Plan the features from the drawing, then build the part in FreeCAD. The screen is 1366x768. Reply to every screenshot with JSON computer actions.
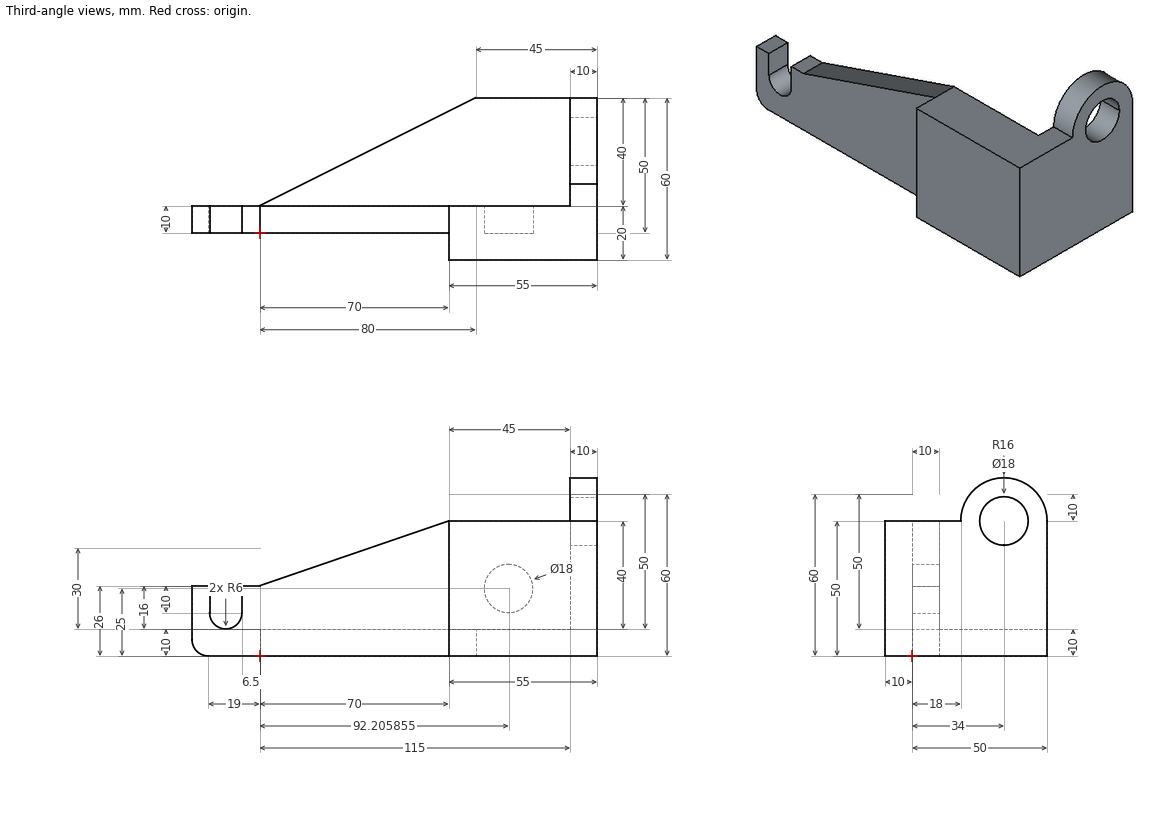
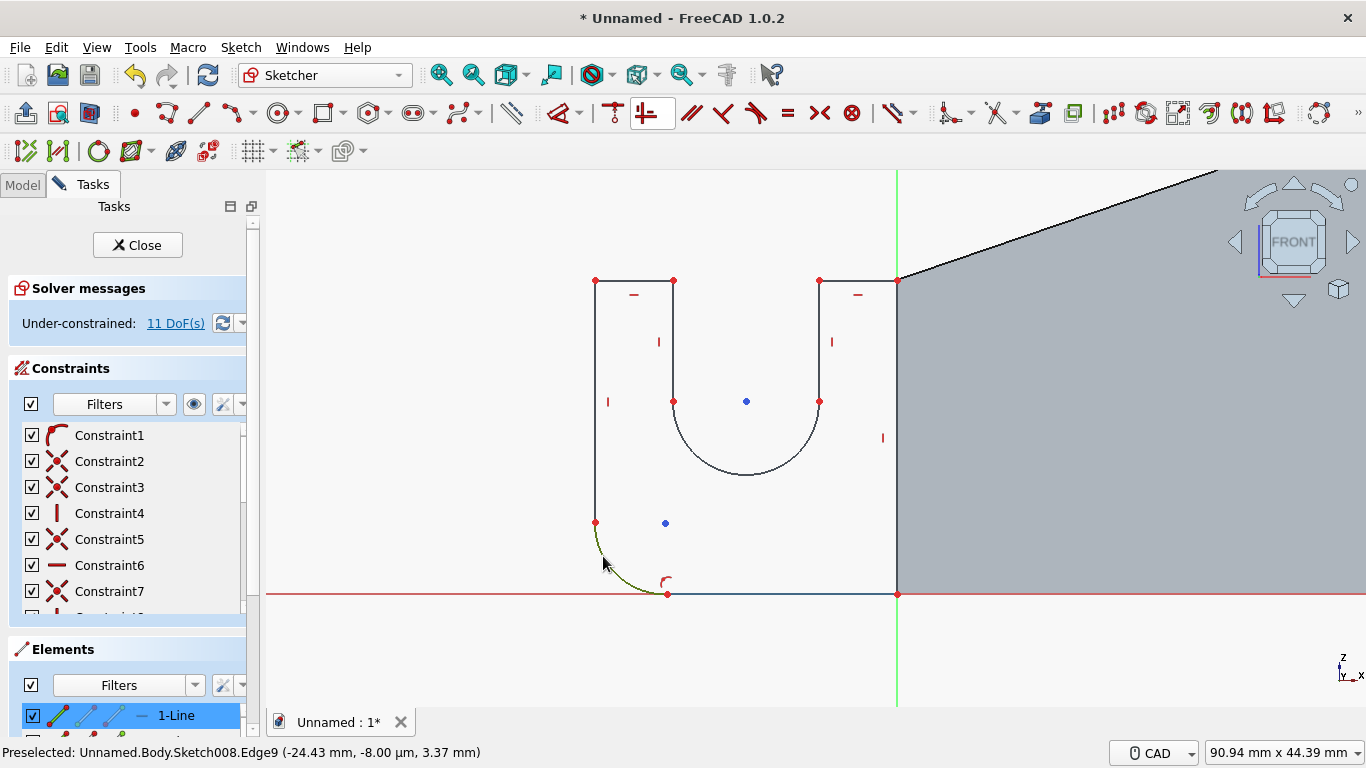
{"action": "left_click", "coordinate": [756, 114]}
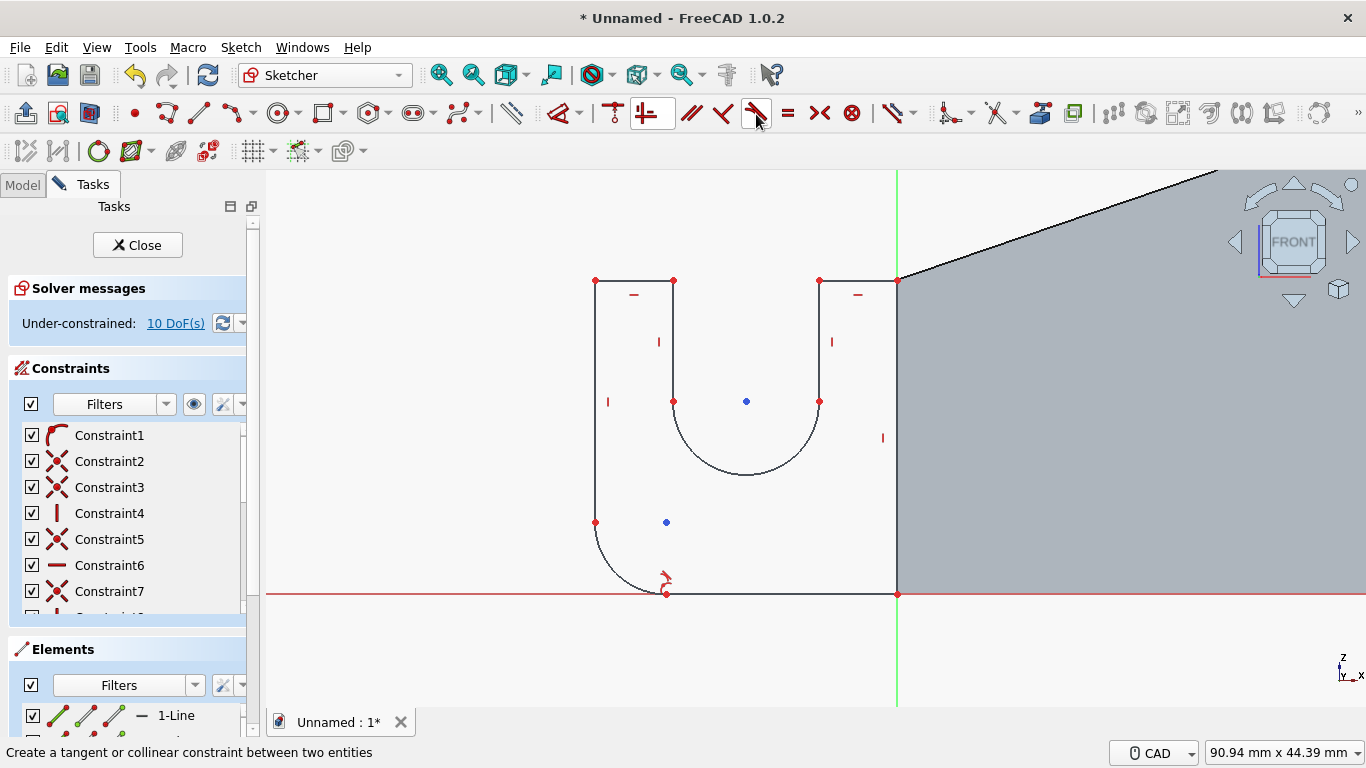
{"action": "left_click", "coordinate": [819, 317]}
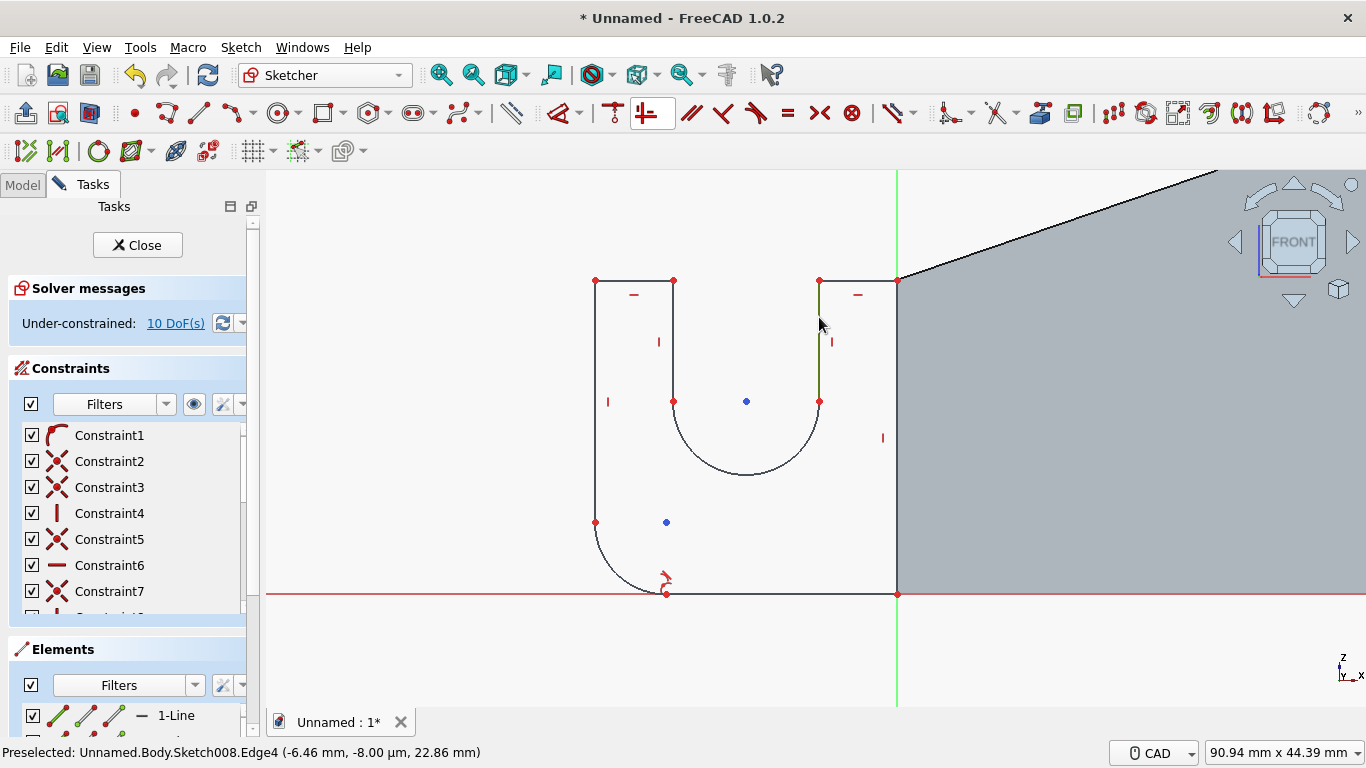
{"action": "left_click", "coordinate": [703, 461]}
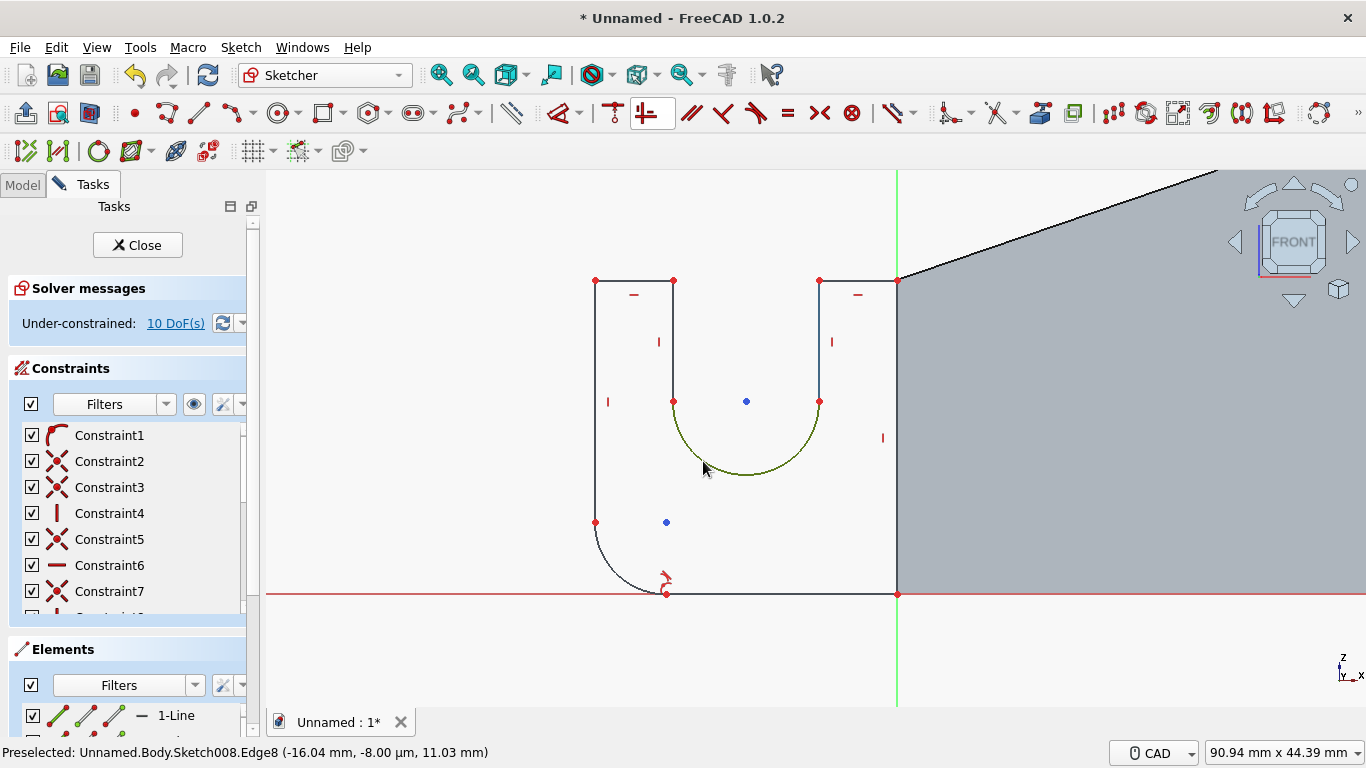
{"action": "left_click", "coordinate": [756, 114]}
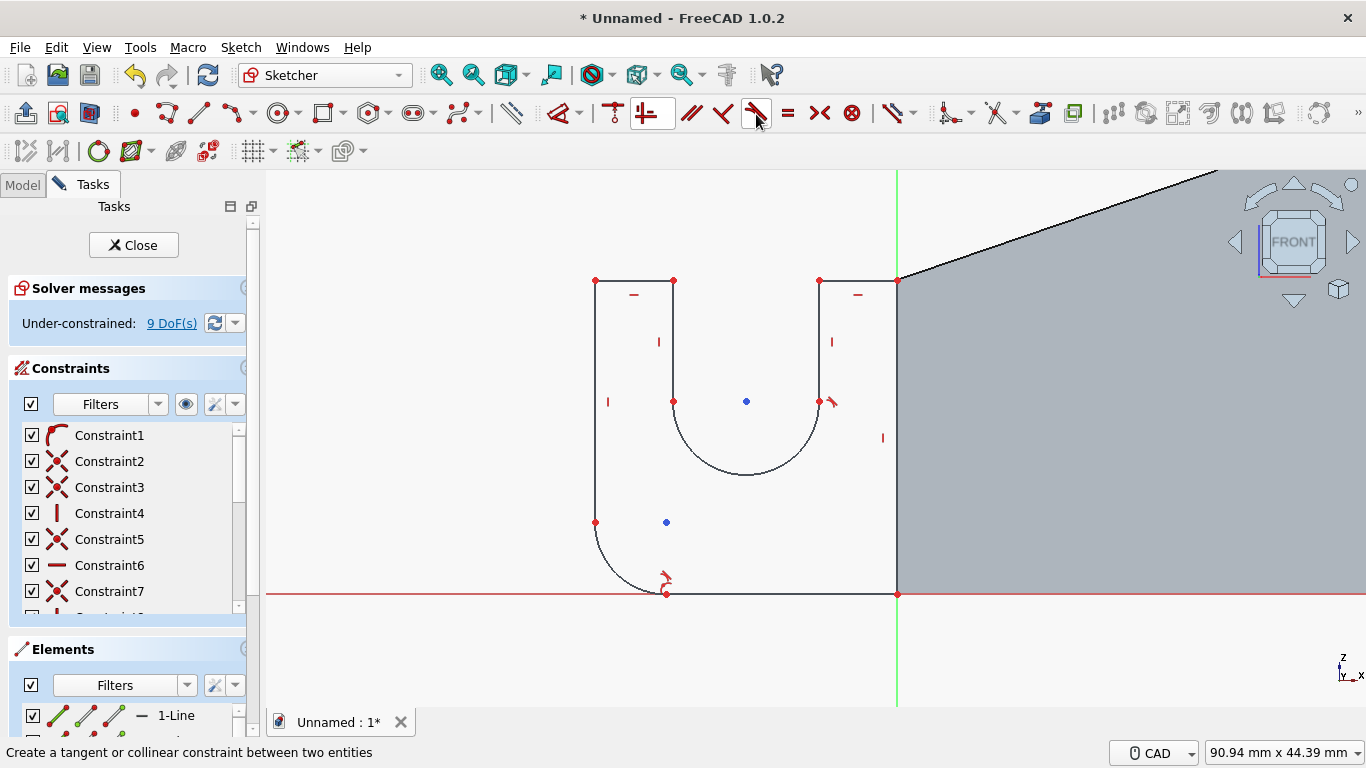
{"action": "left_click", "coordinate": [673, 366]}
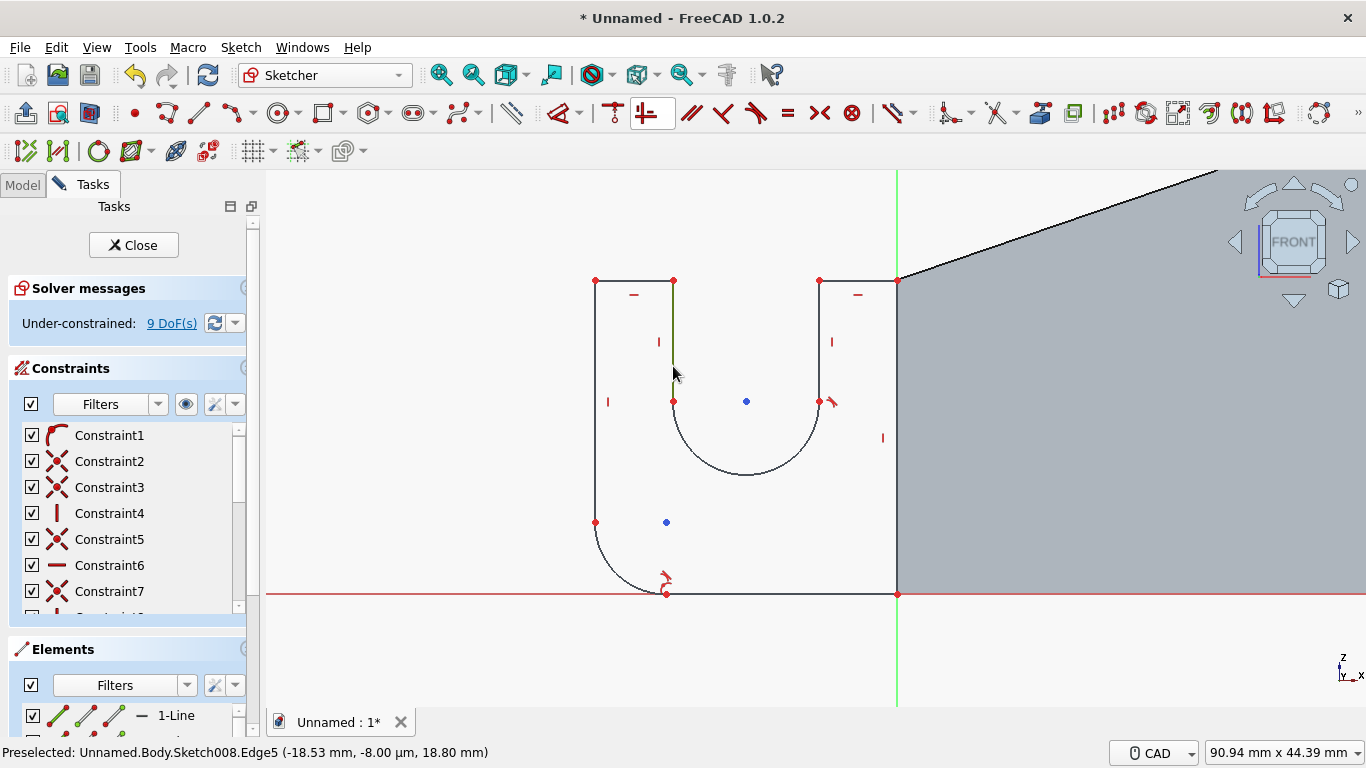
{"action": "left_click", "coordinate": [703, 461]}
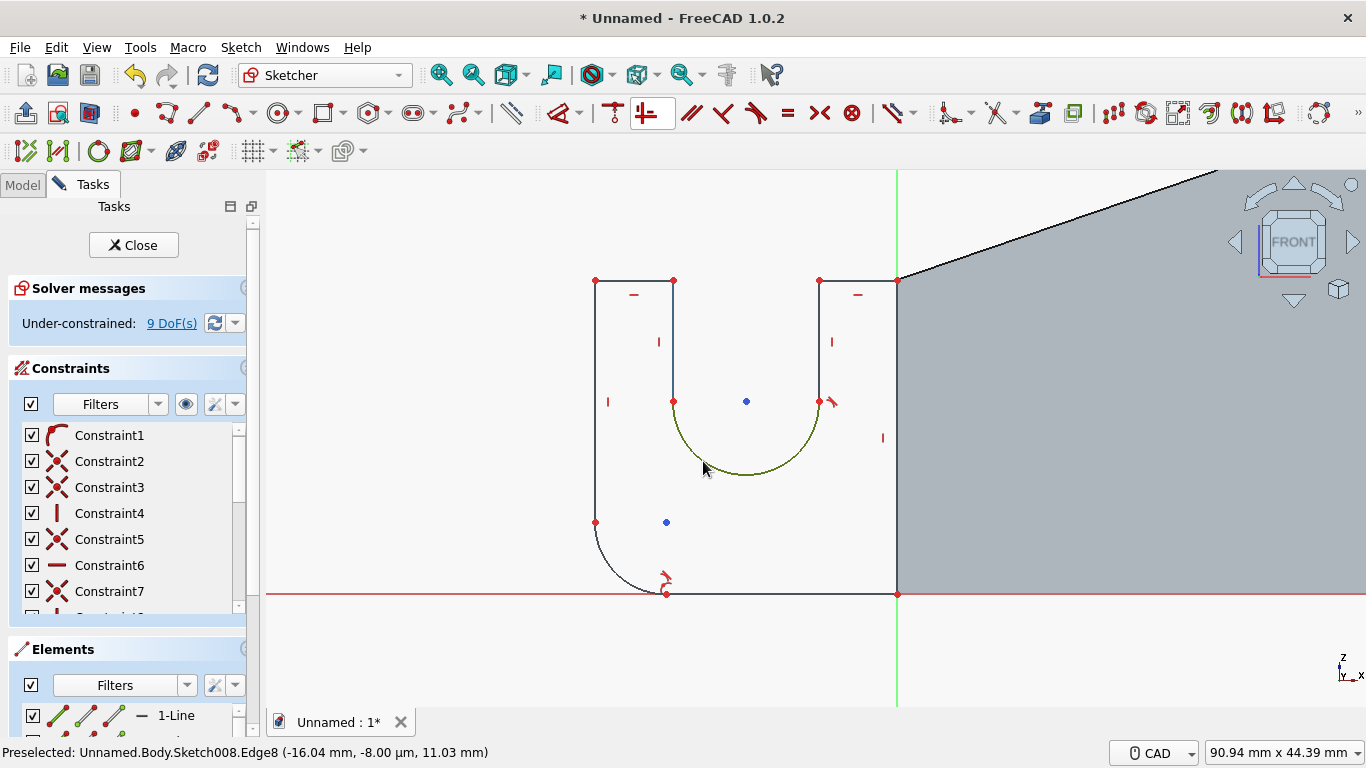
{"action": "left_click", "coordinate": [756, 114]}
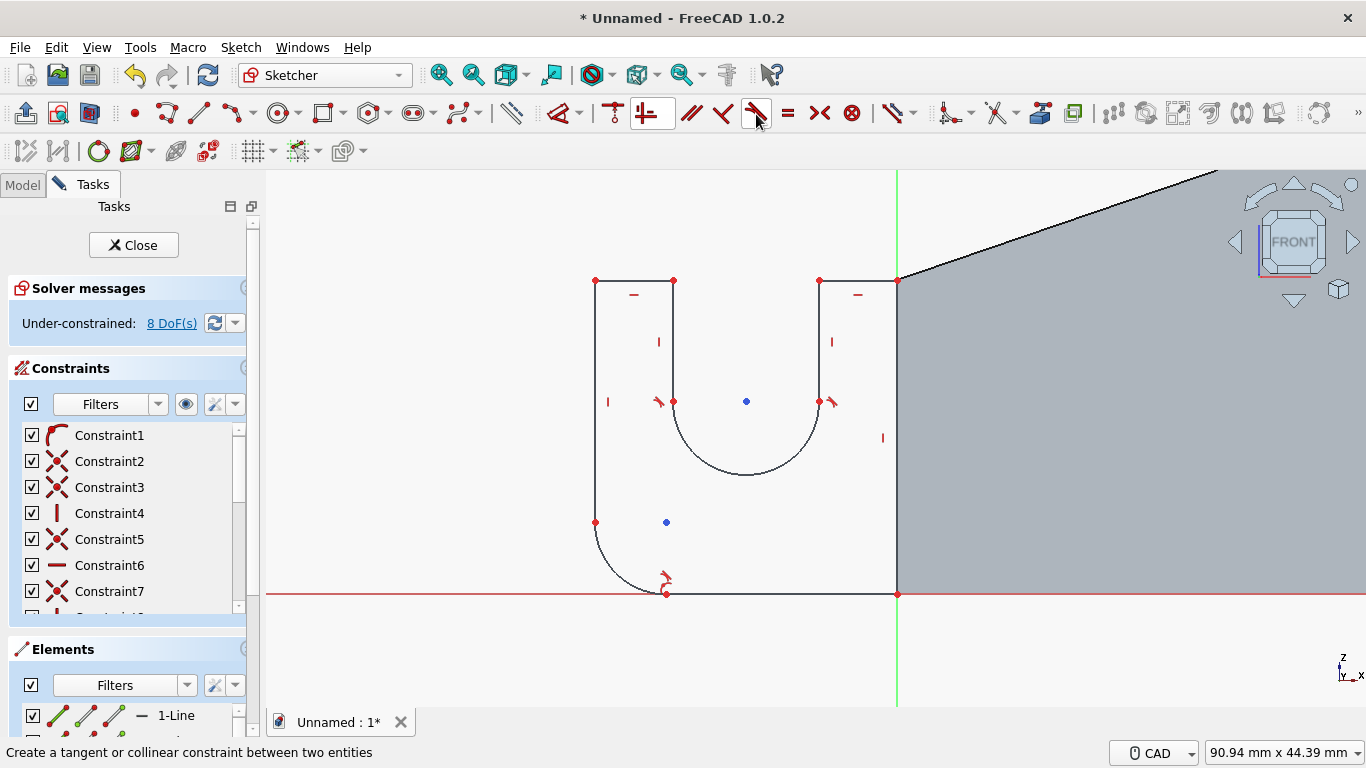
{"action": "left_click", "coordinate": [595, 354]}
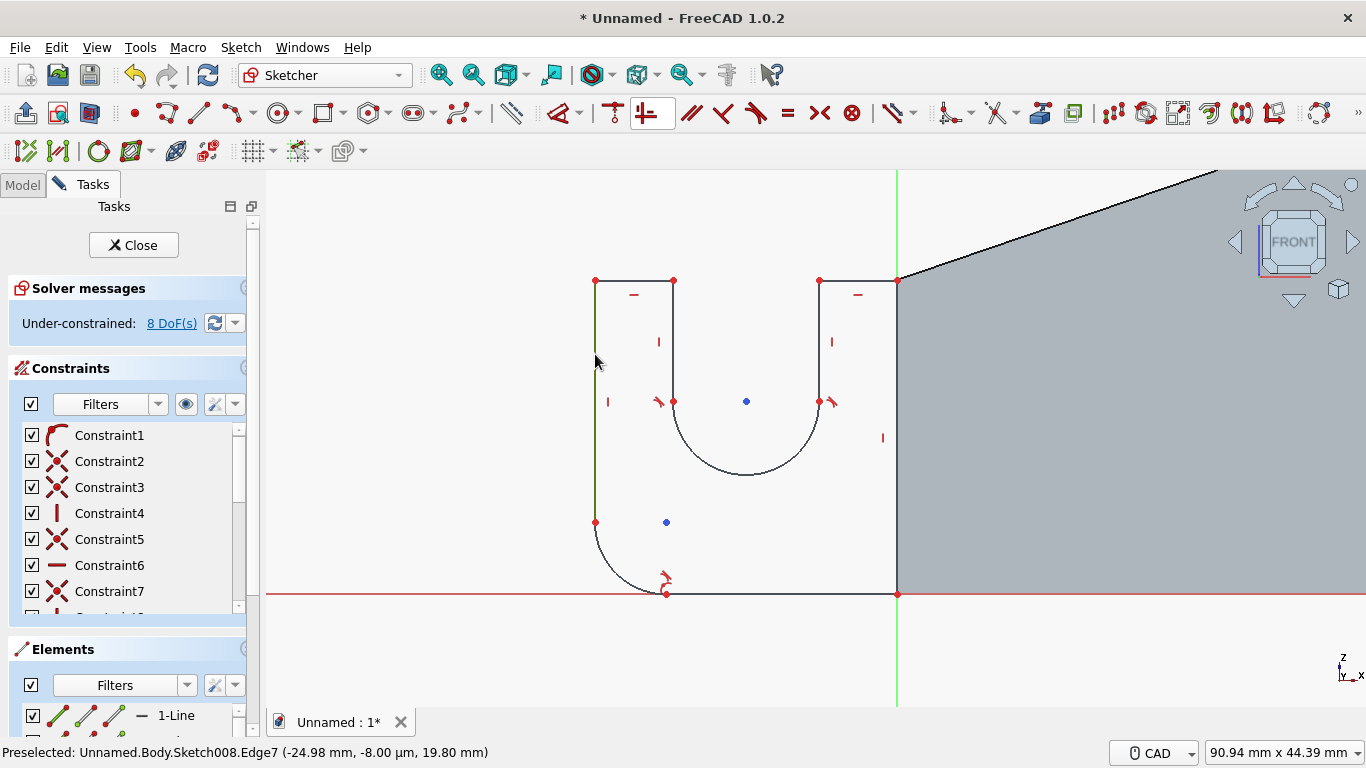
{"action": "left_click", "coordinate": [603, 555]}